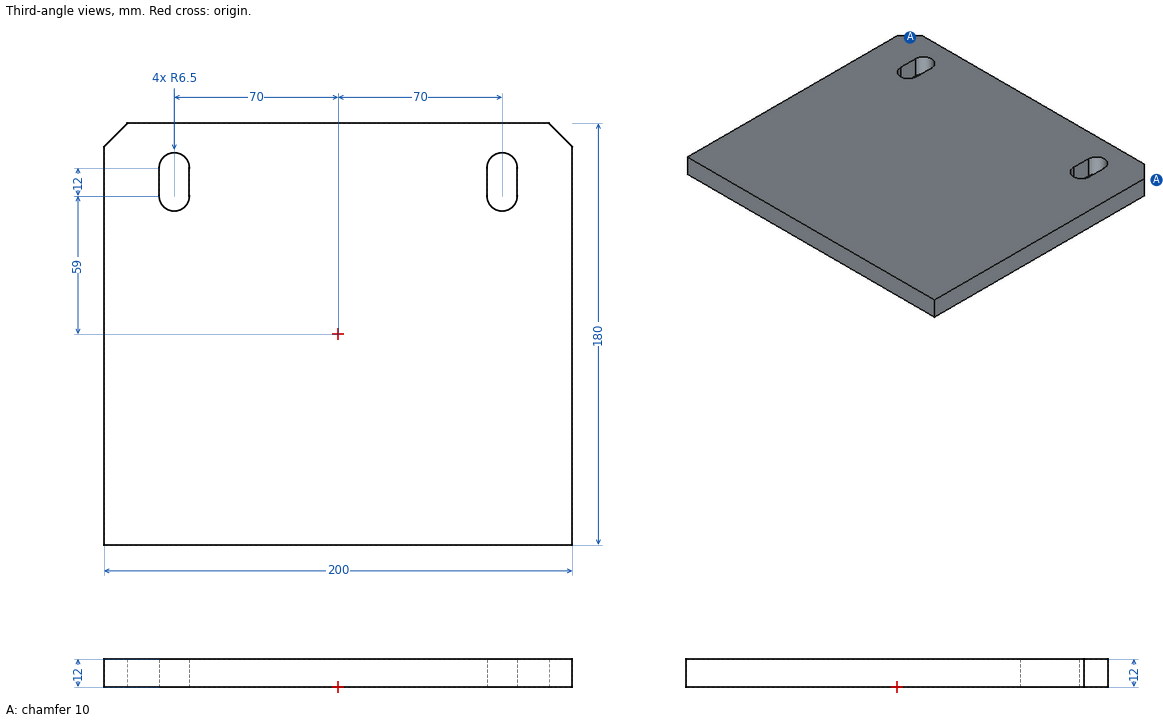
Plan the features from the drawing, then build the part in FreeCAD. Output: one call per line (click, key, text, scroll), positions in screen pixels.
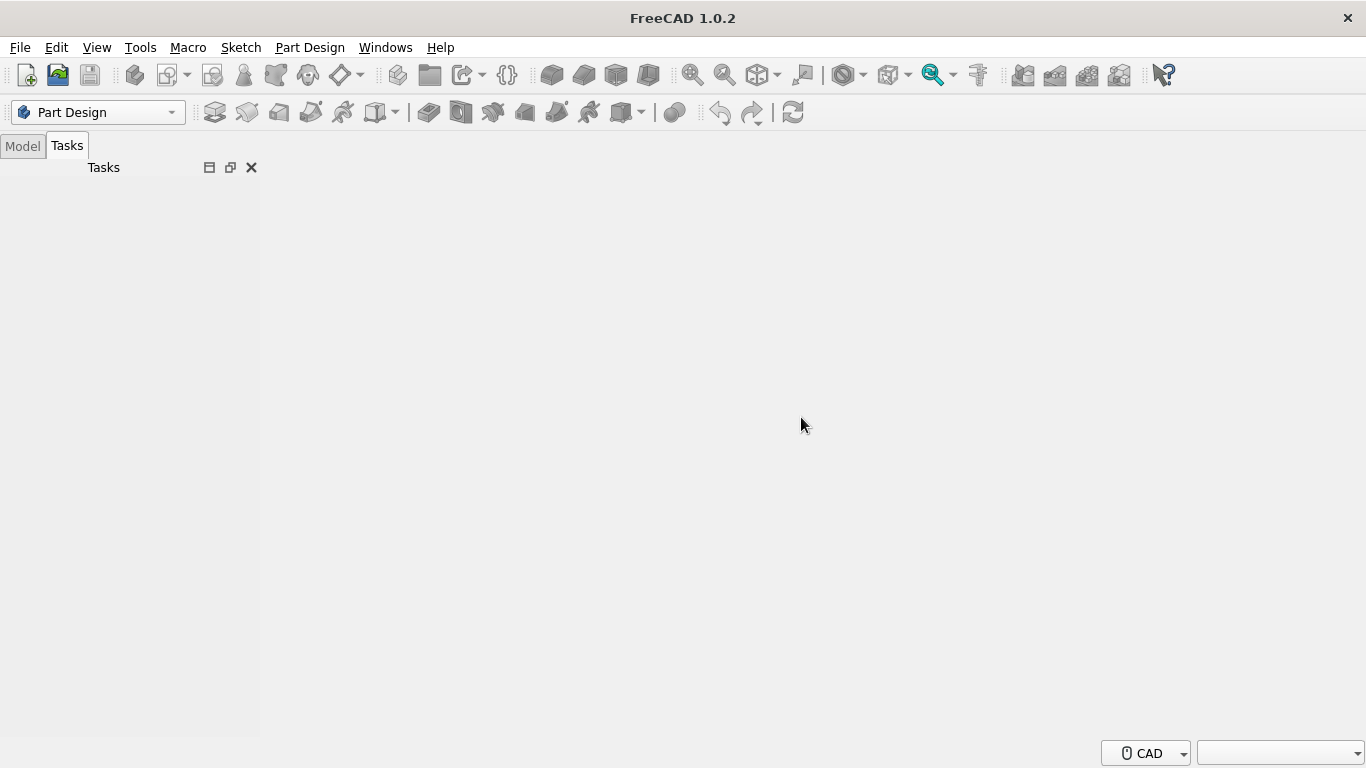
key(ctrl+n)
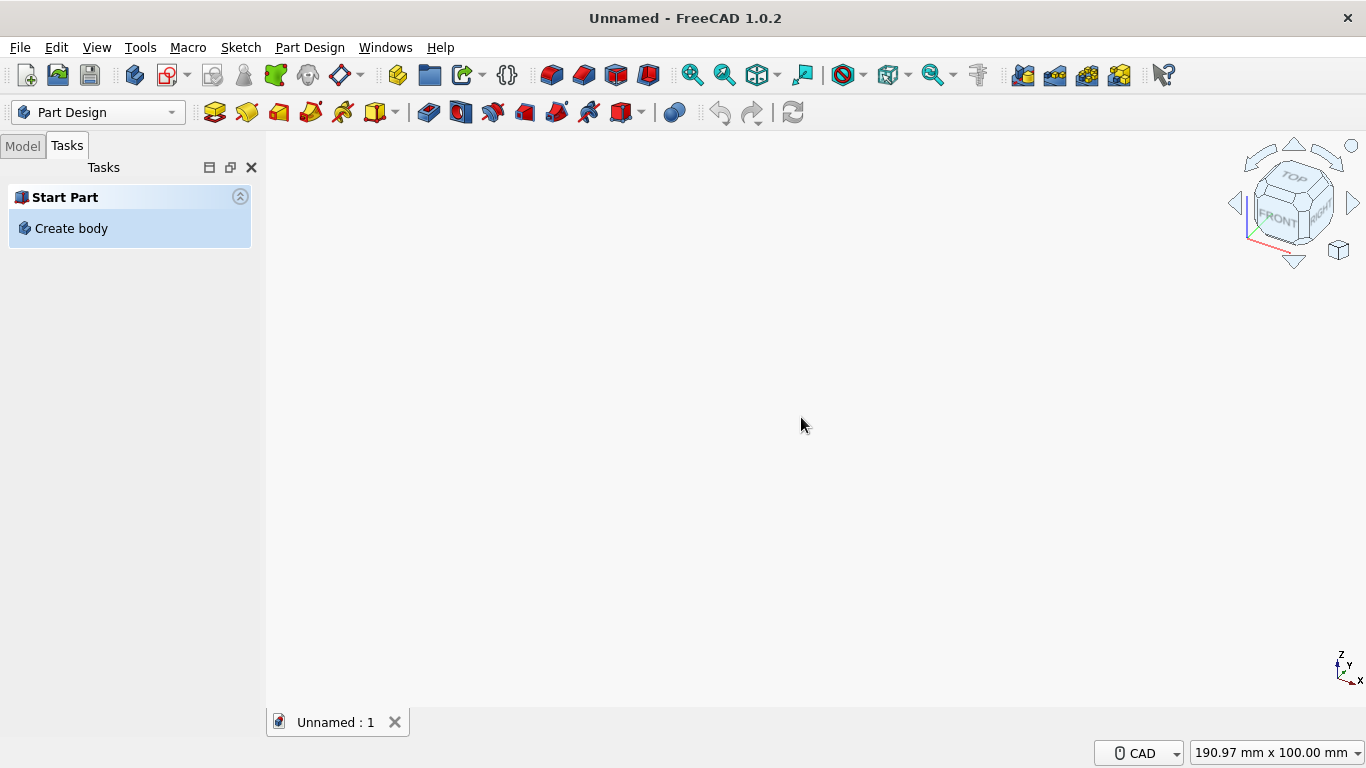
click(168, 76)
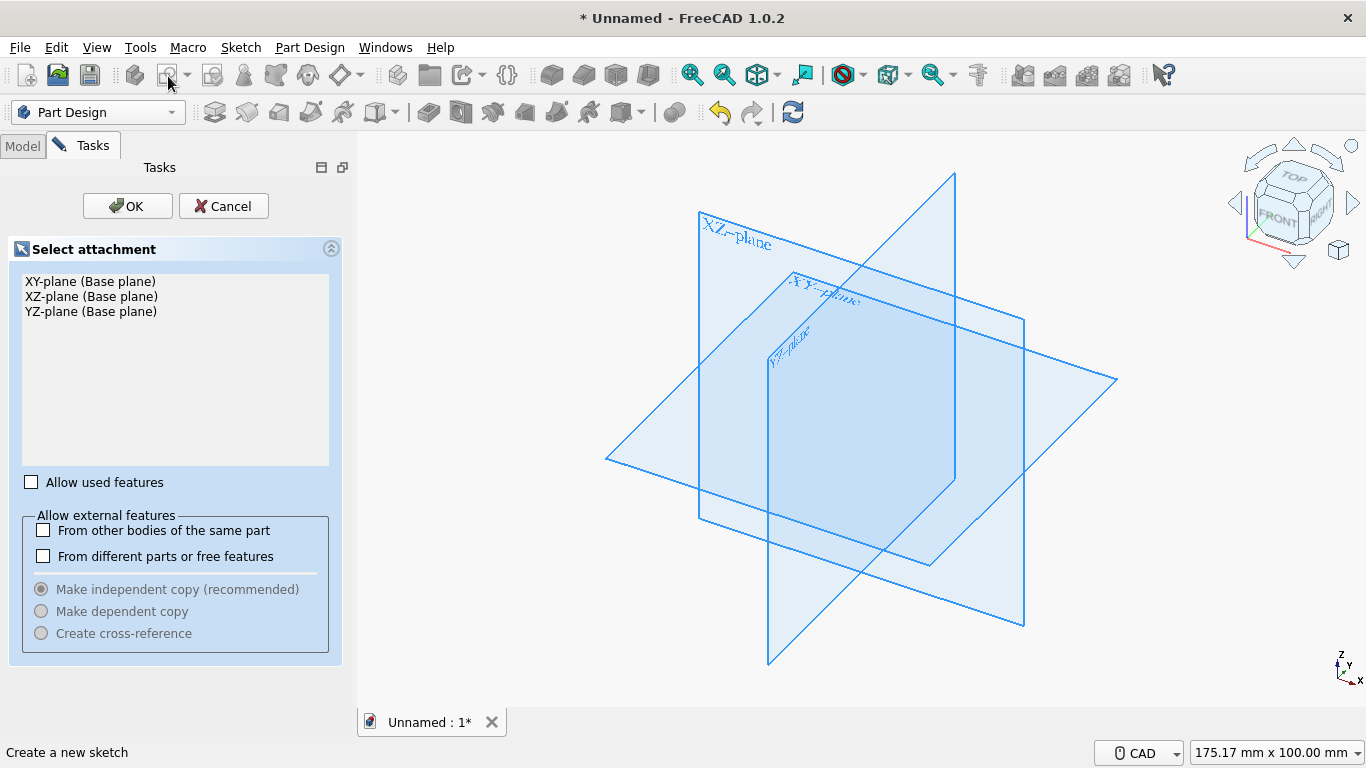
click(82, 282)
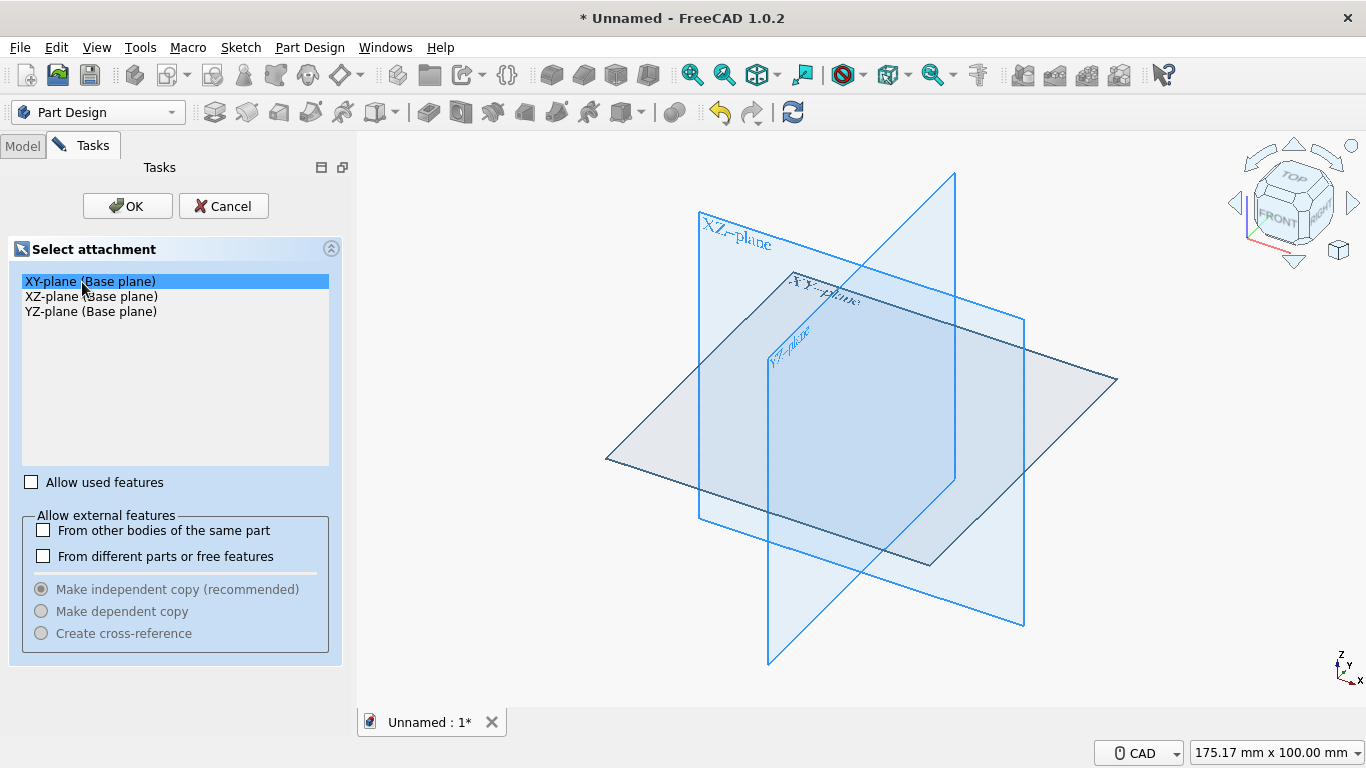
click(128, 206)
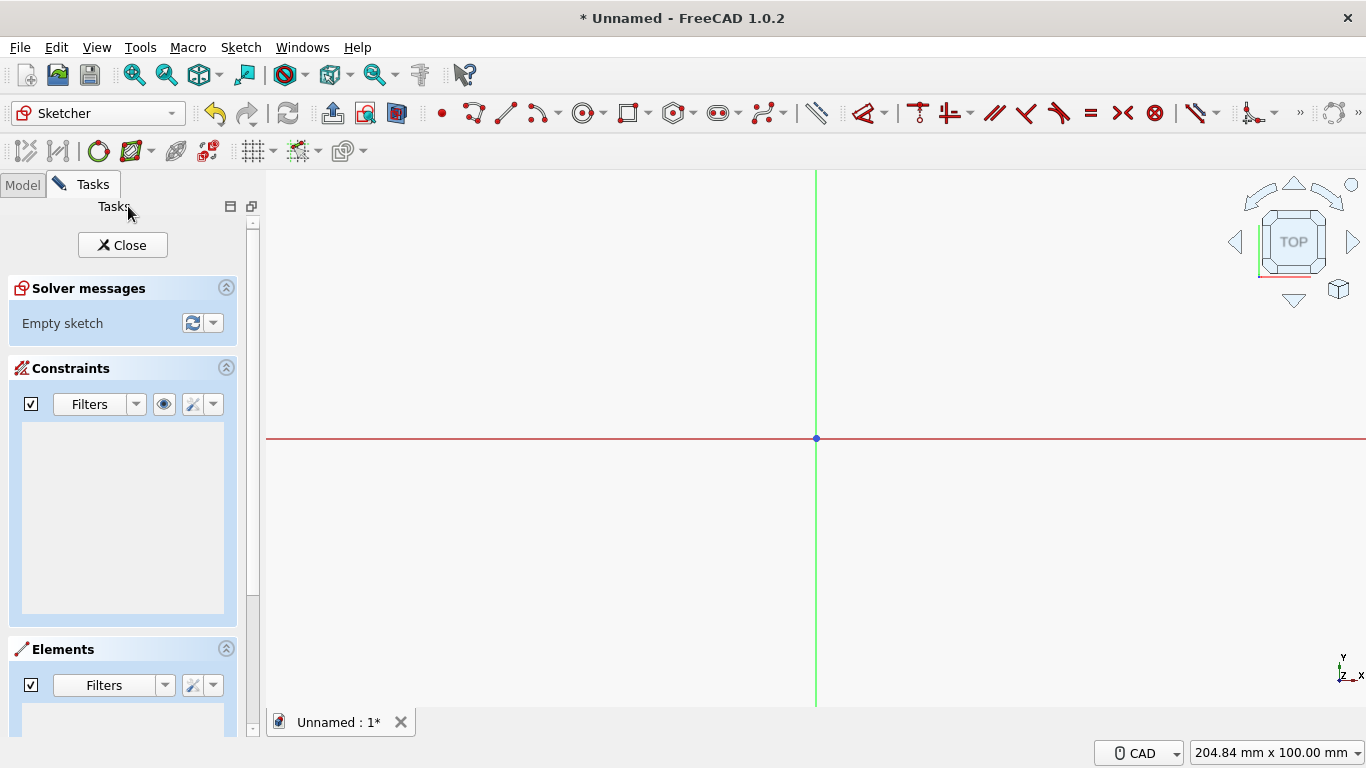
scroll(708, 439, down, 5)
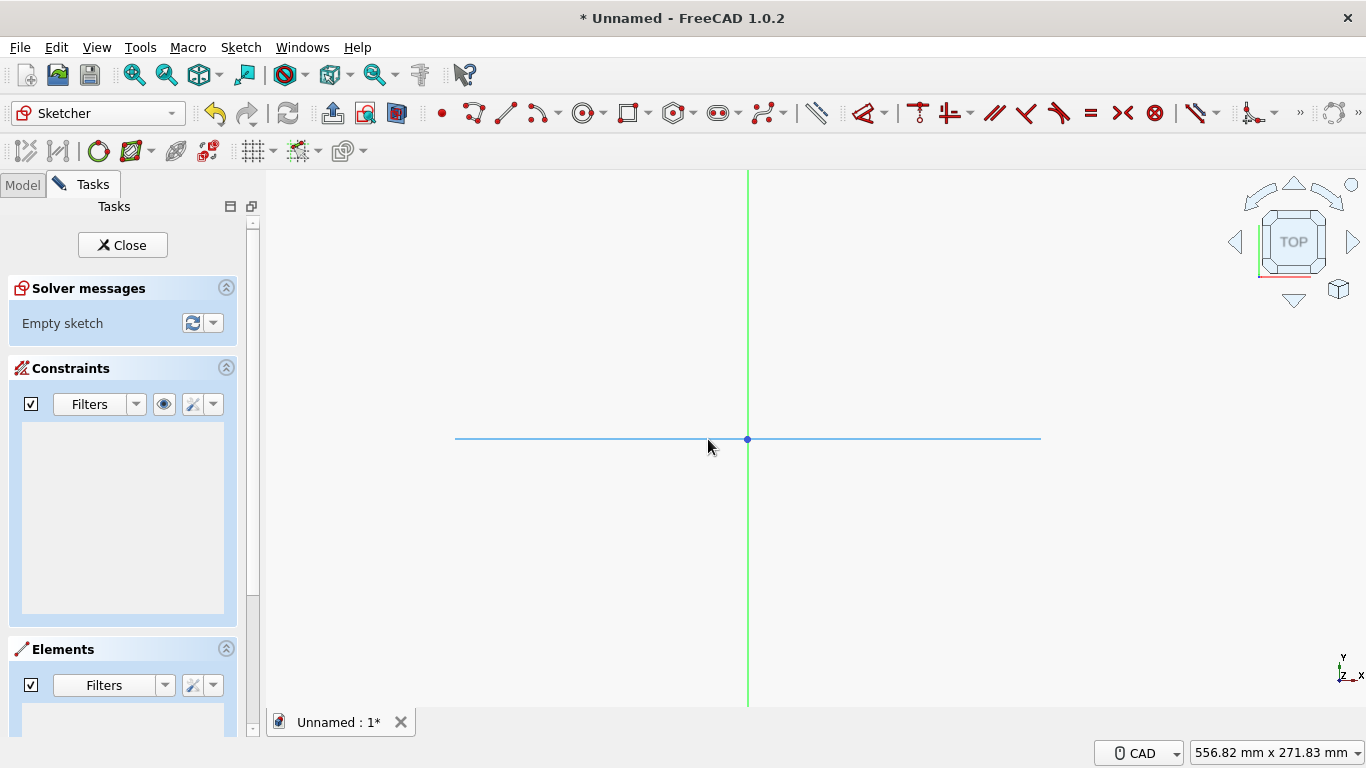
key(g)
key(v)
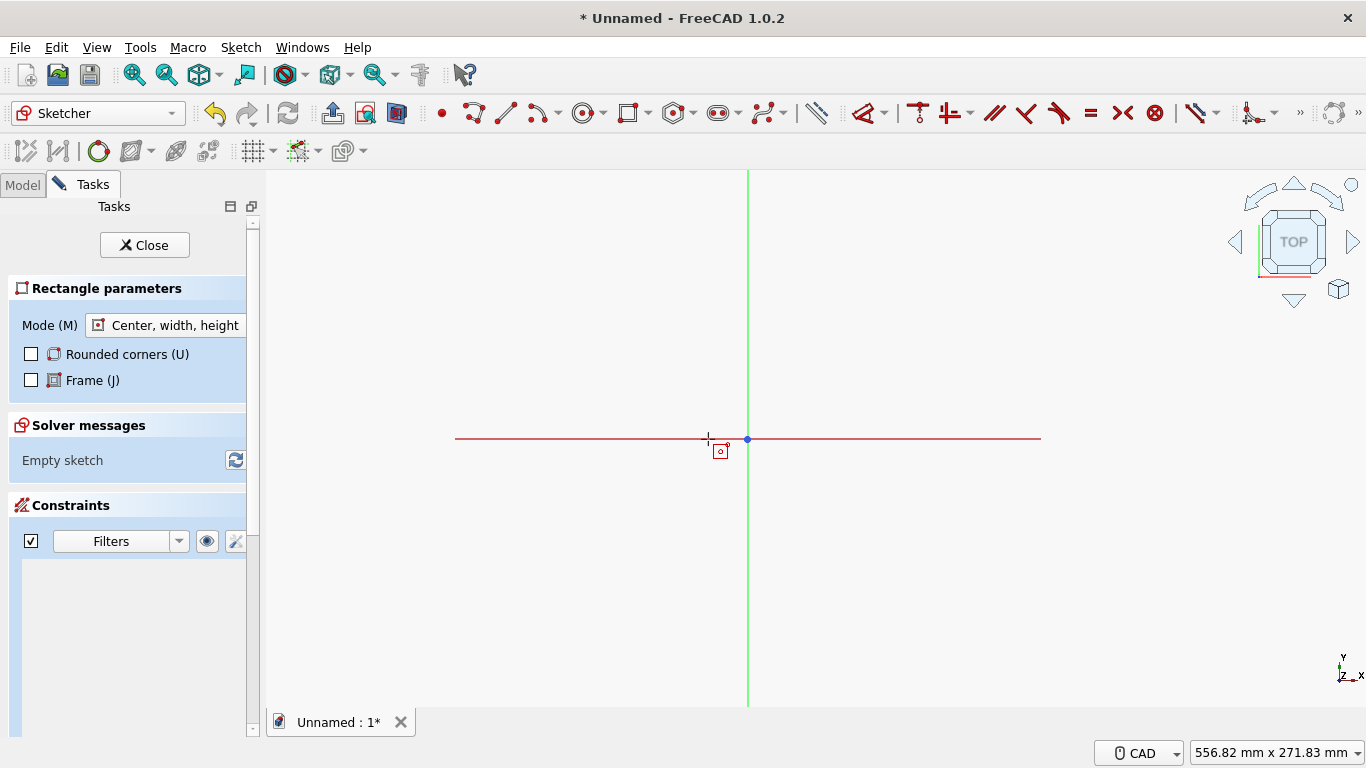
click(748, 439)
click(946, 261)
key(Escape)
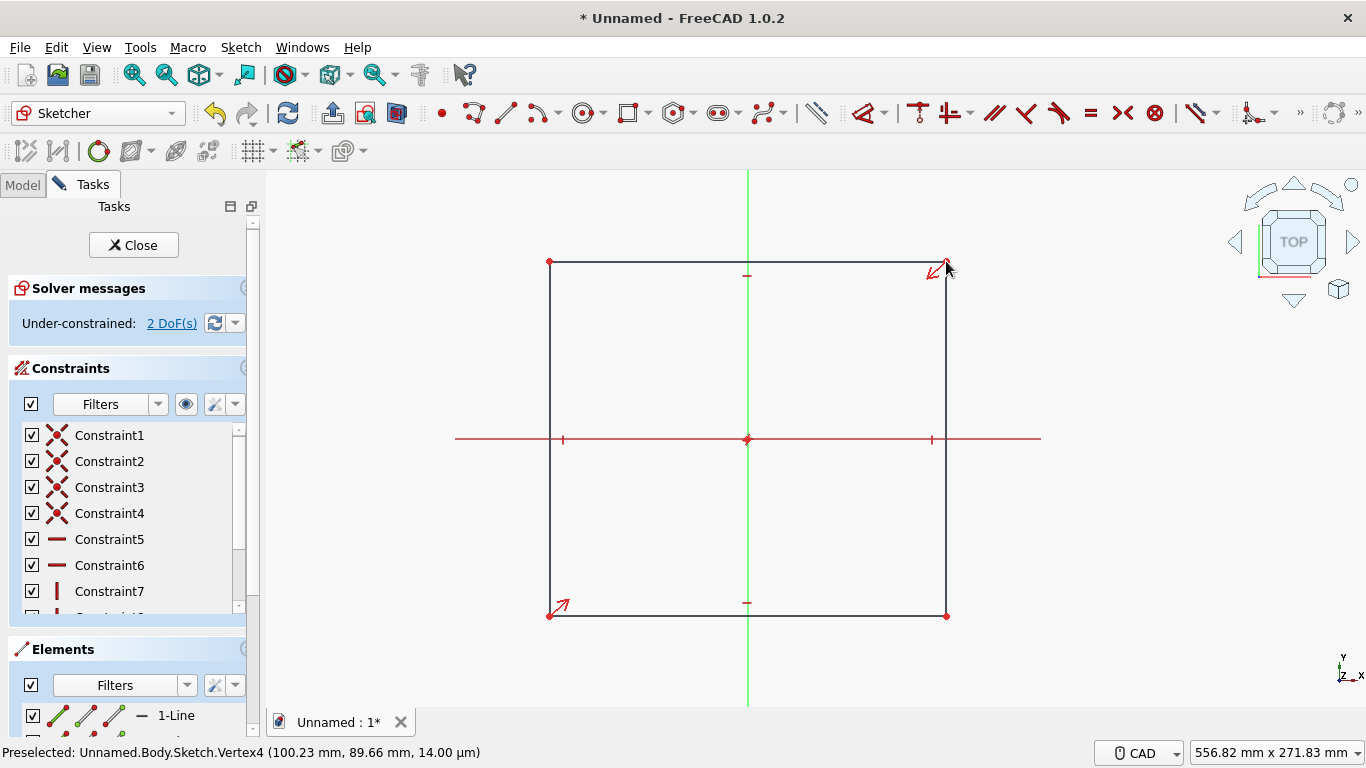
click(669, 616)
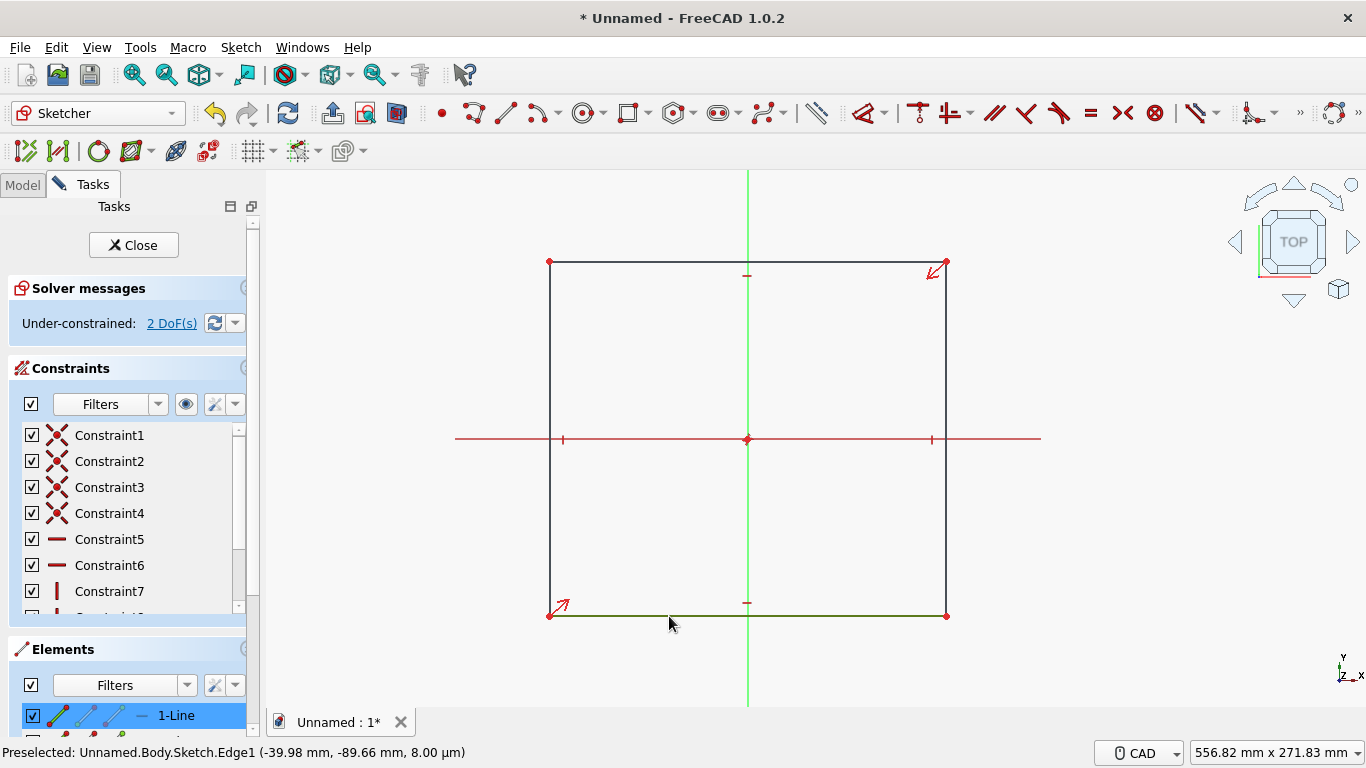
key(l)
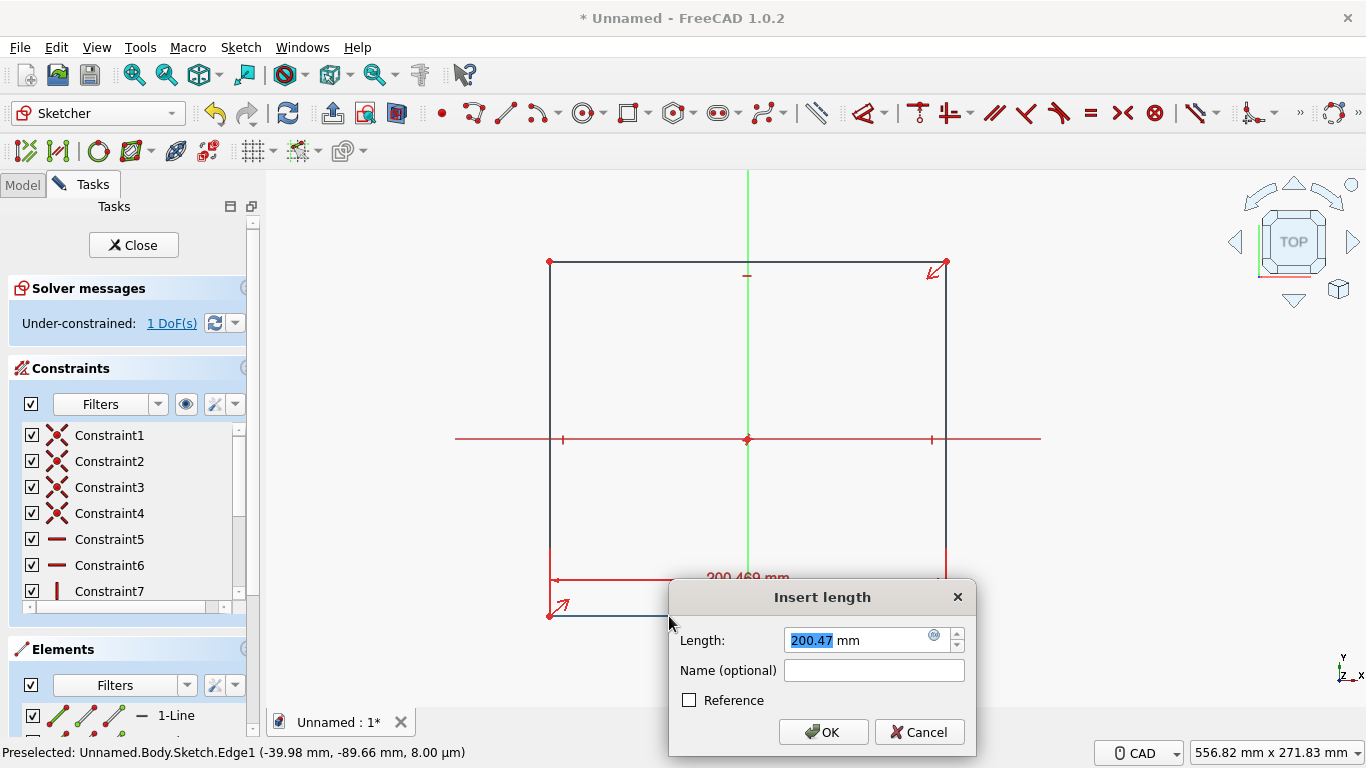
text(200)
key(Return)